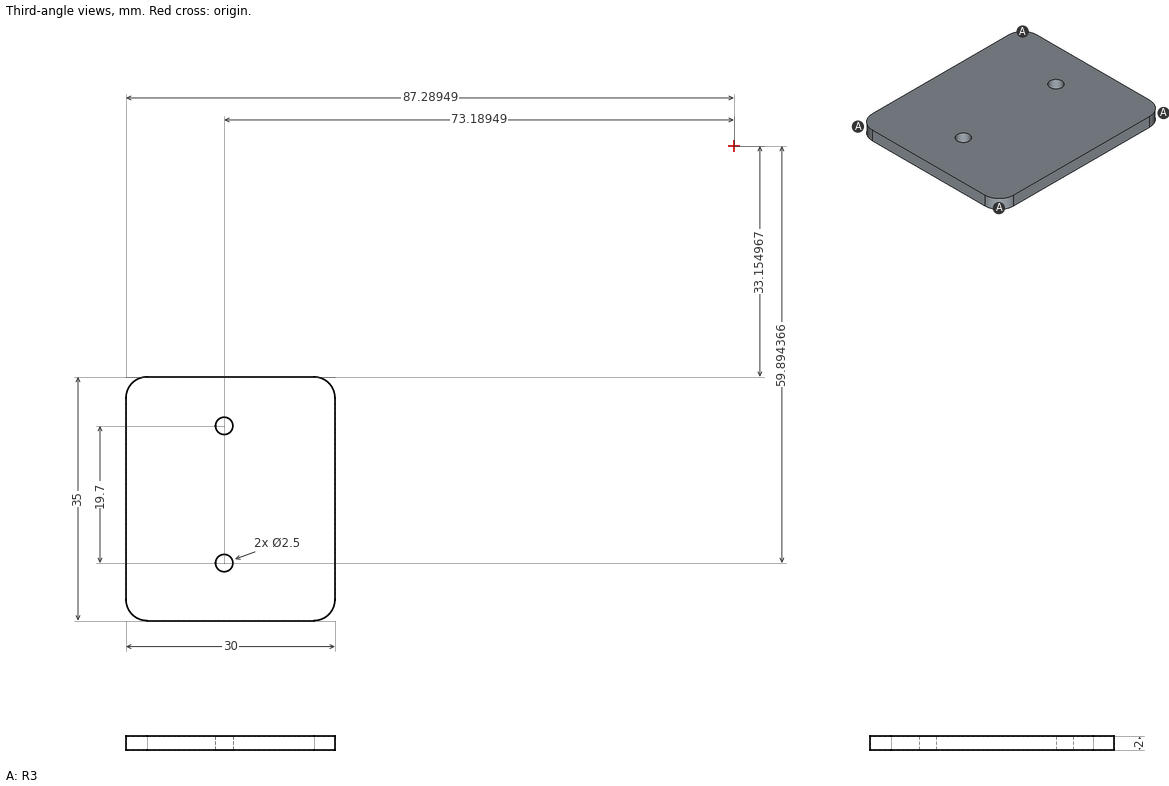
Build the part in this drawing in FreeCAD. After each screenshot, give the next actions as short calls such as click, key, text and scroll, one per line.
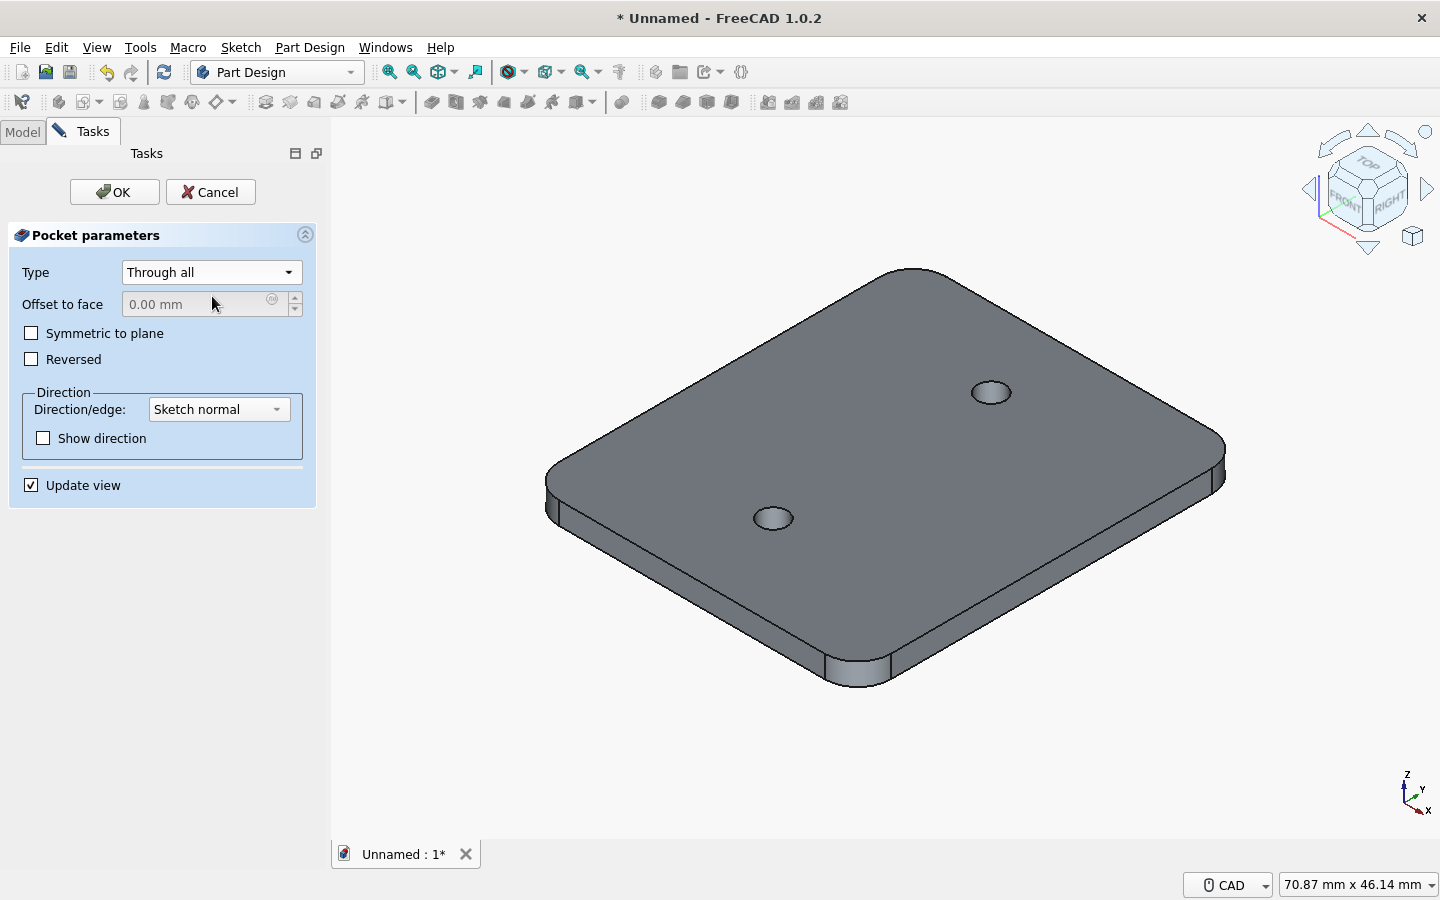
click(115, 192)